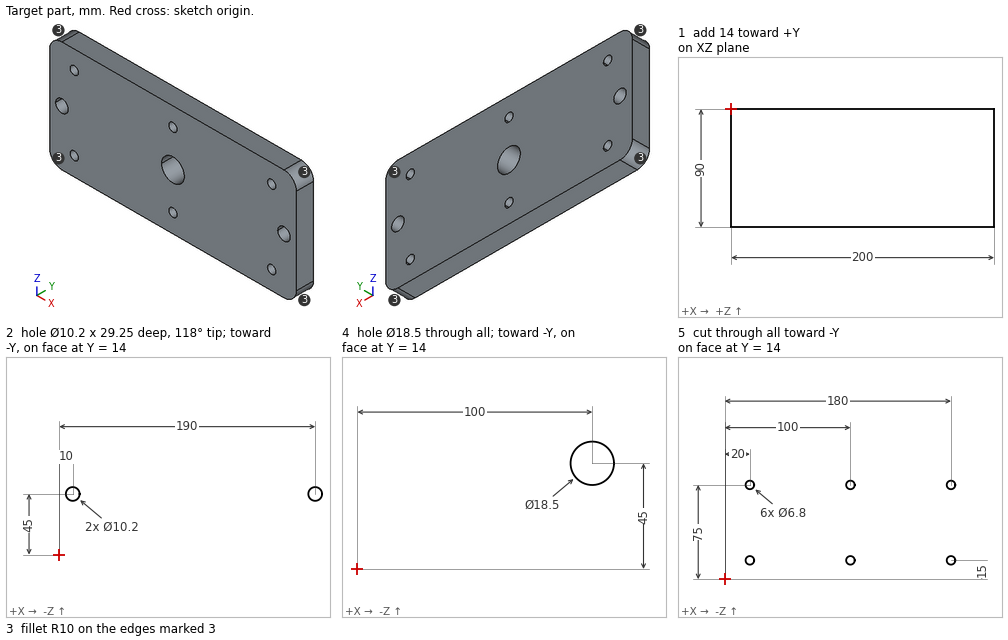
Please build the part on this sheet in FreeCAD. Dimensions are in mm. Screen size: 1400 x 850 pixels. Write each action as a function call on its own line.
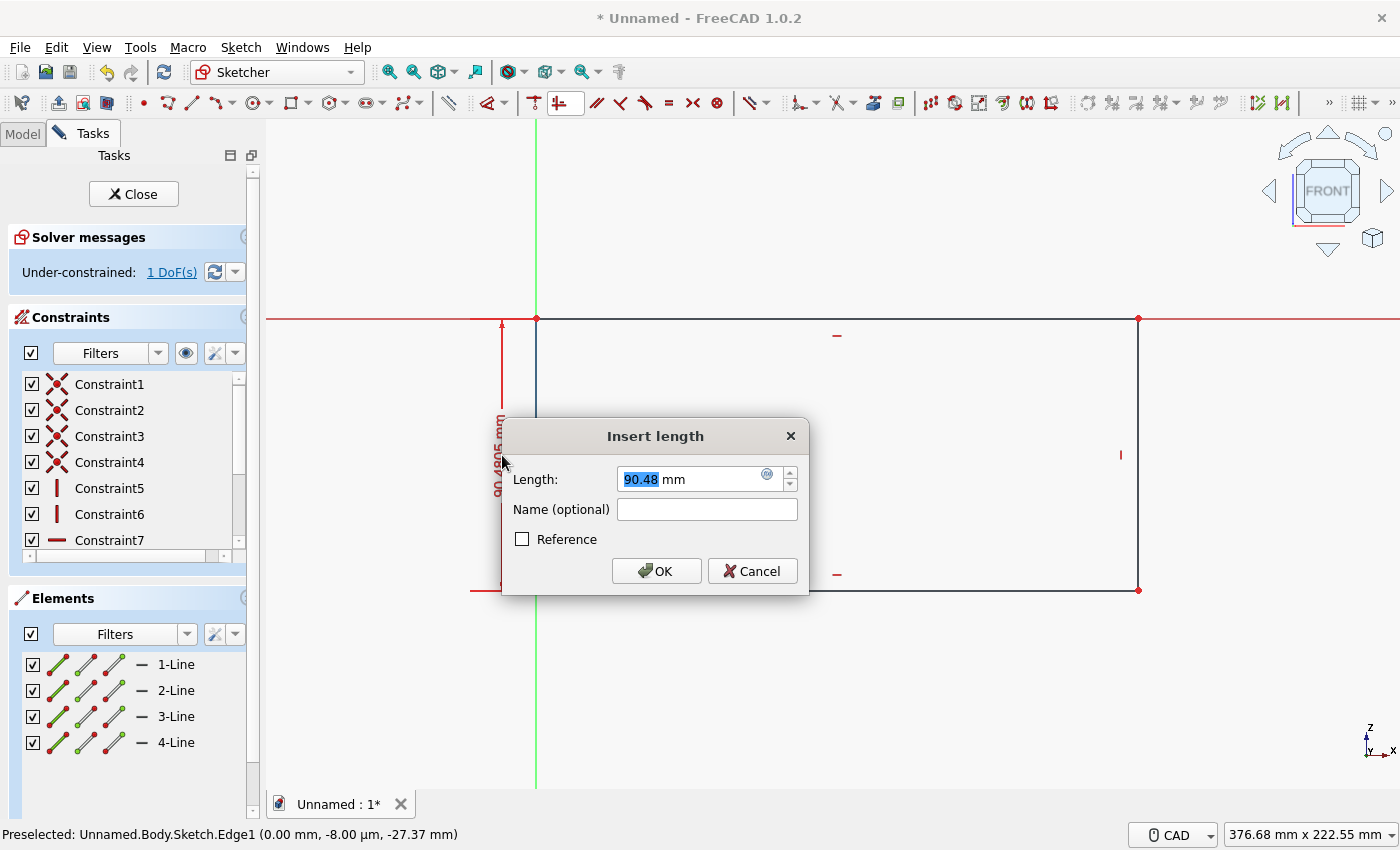
text(90)
key(Return)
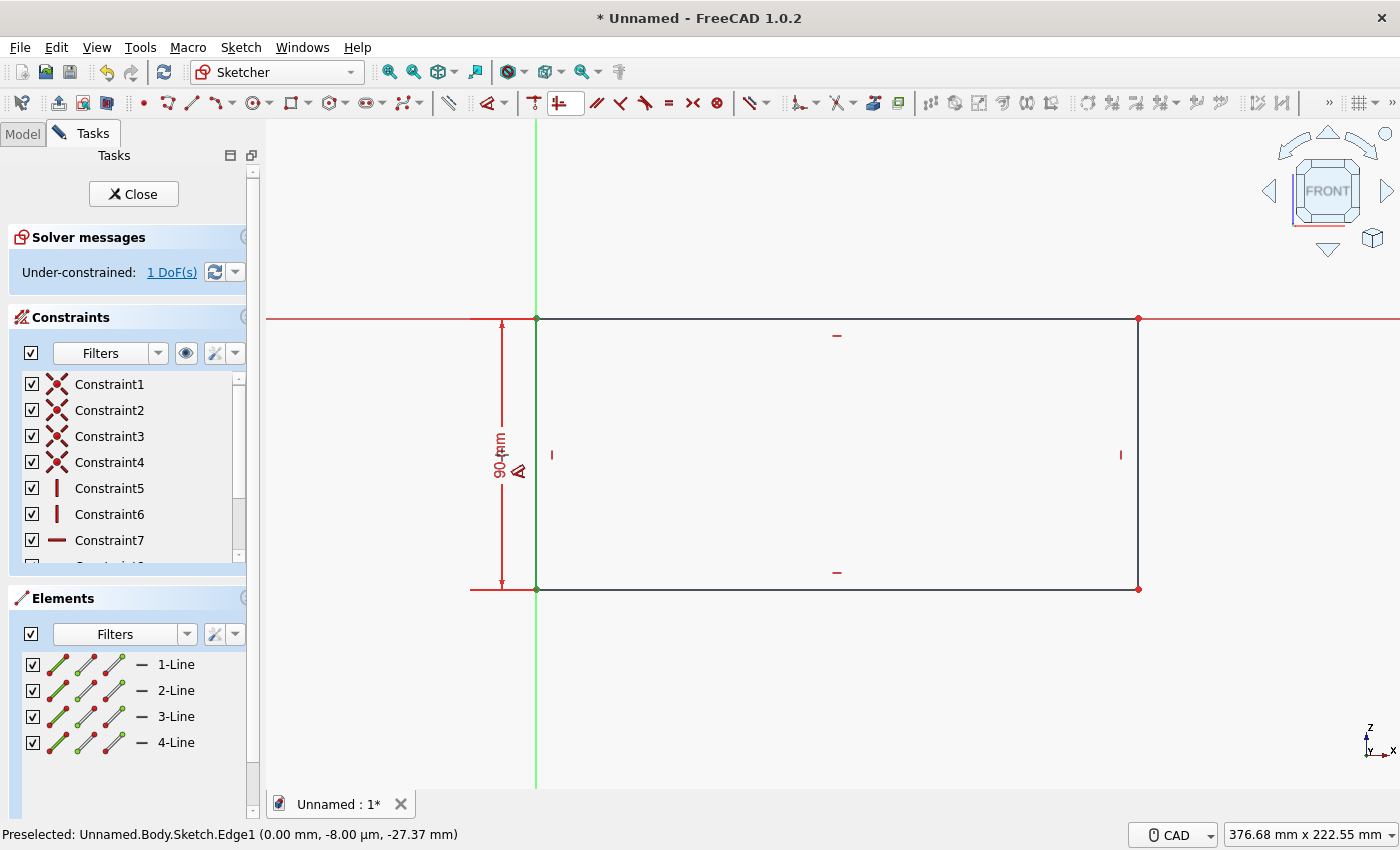
click(717, 590)
click(837, 624)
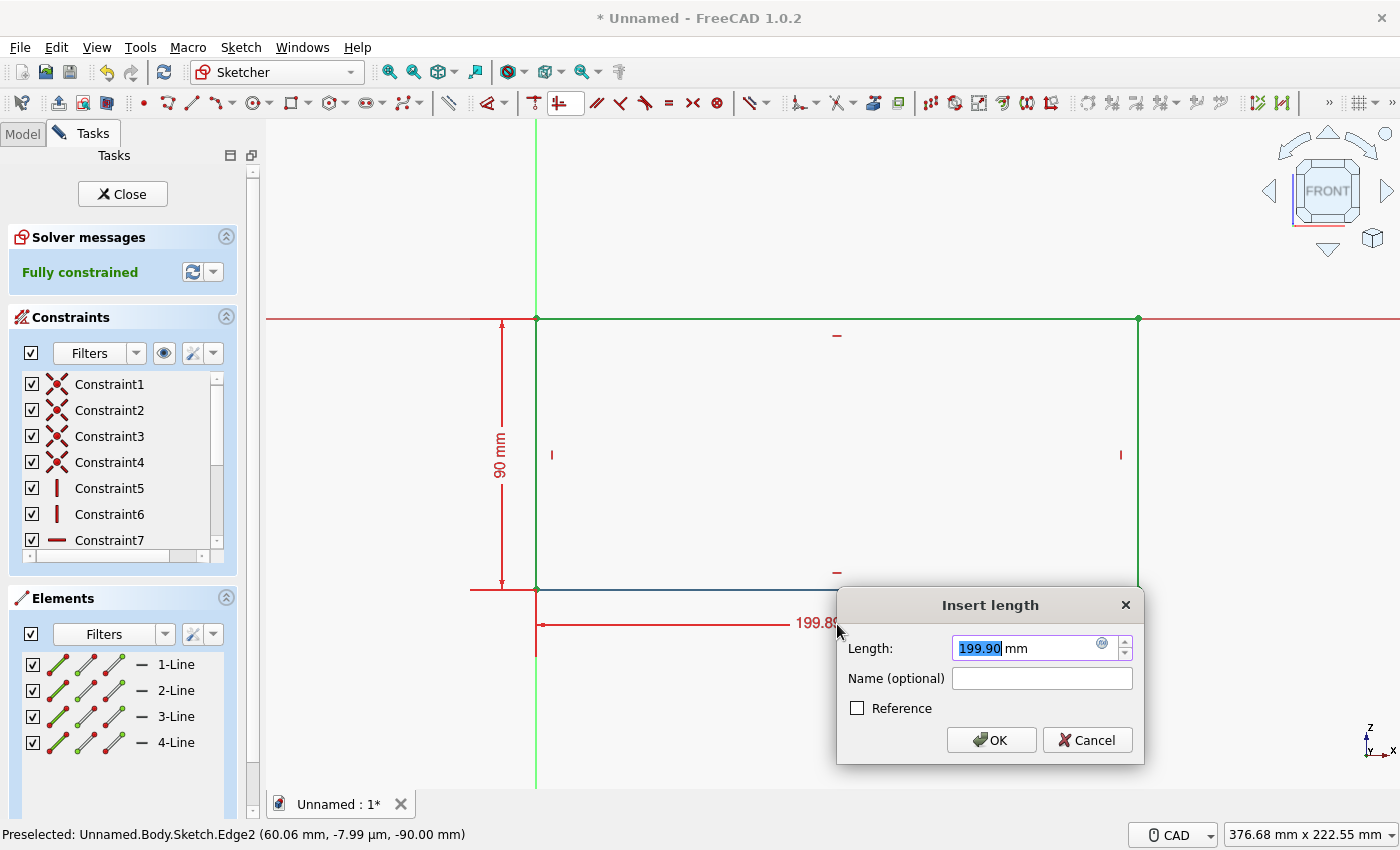
text(200)
key(Return)
key(Escape)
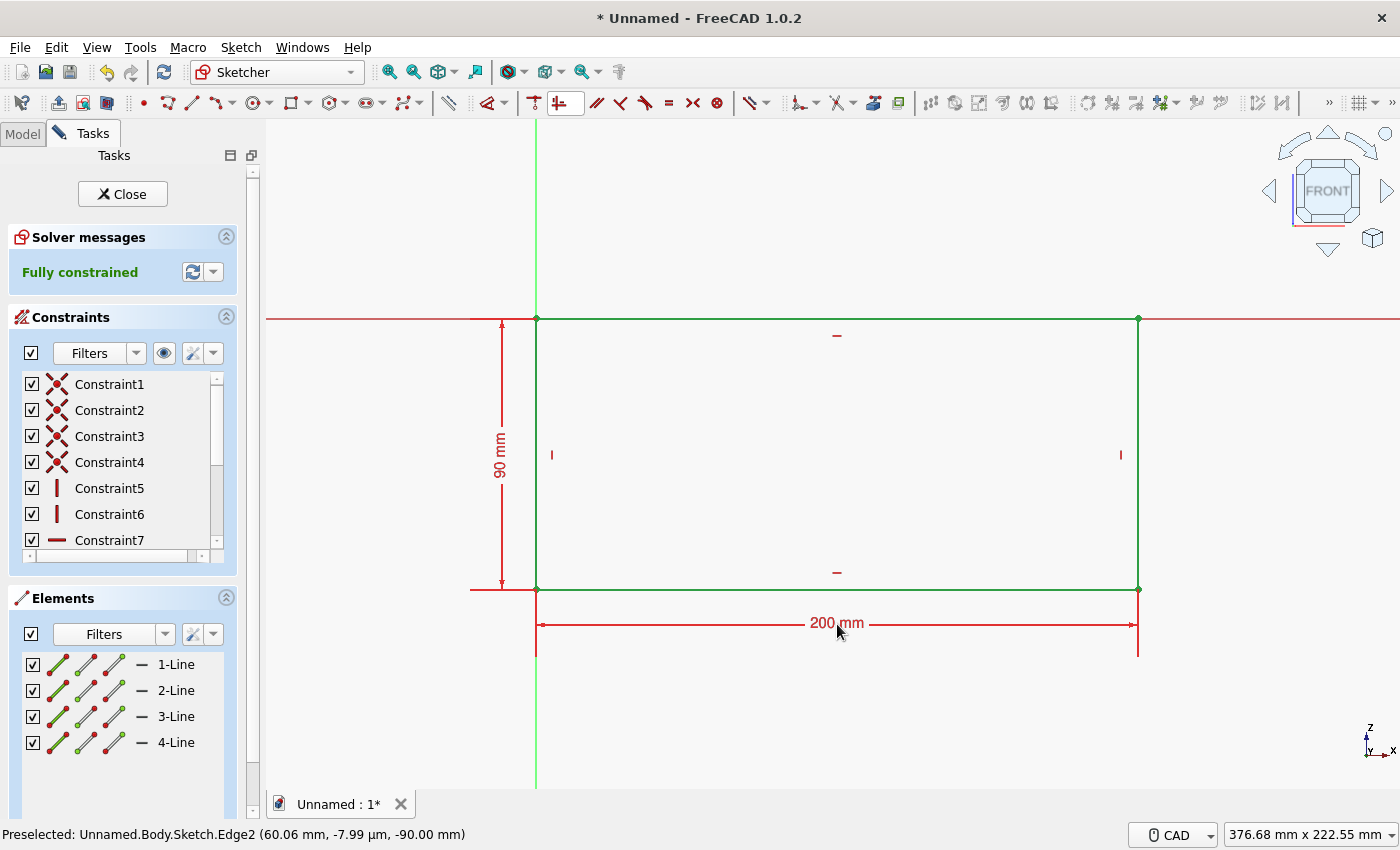
click(123, 194)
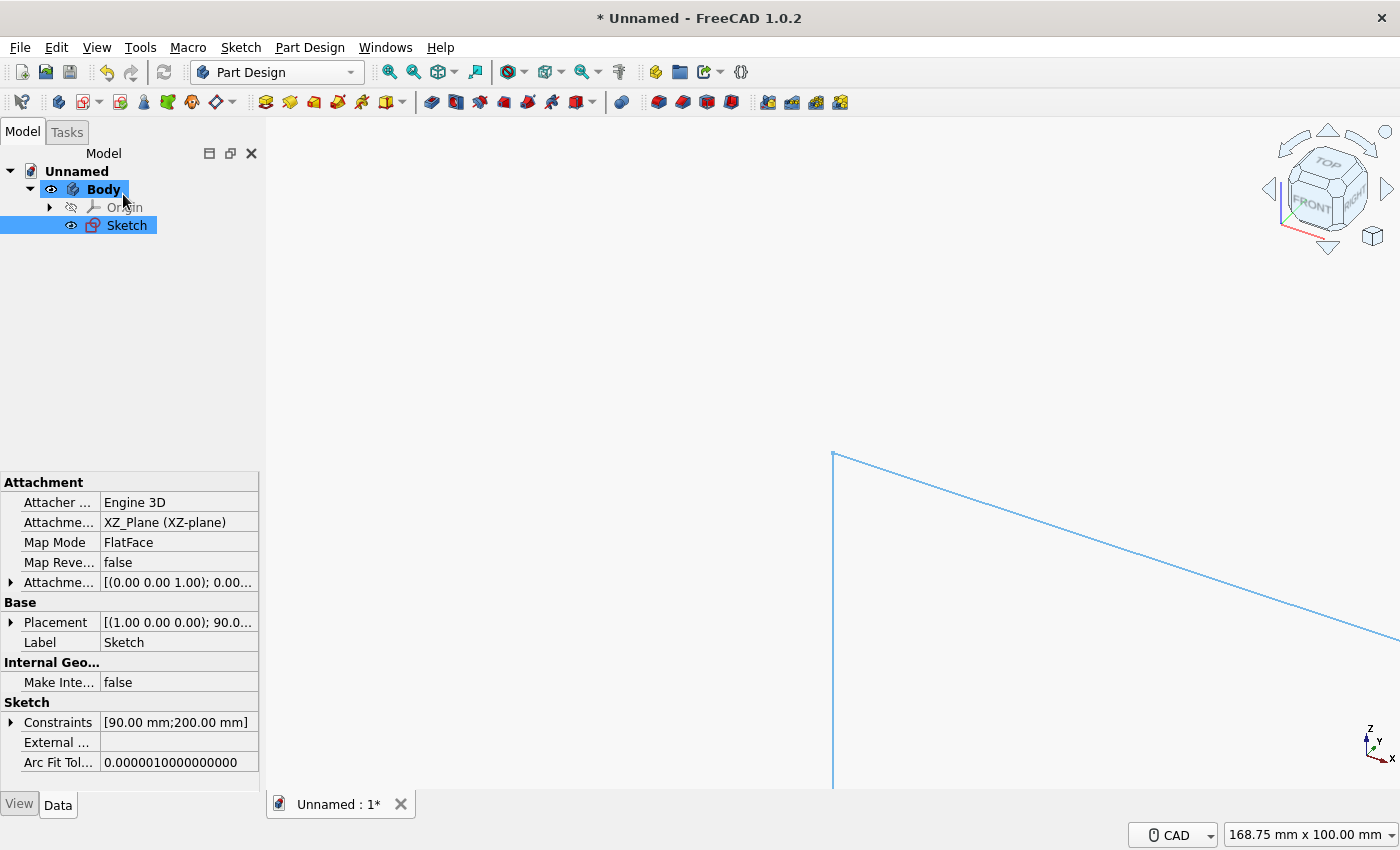
click(266, 102)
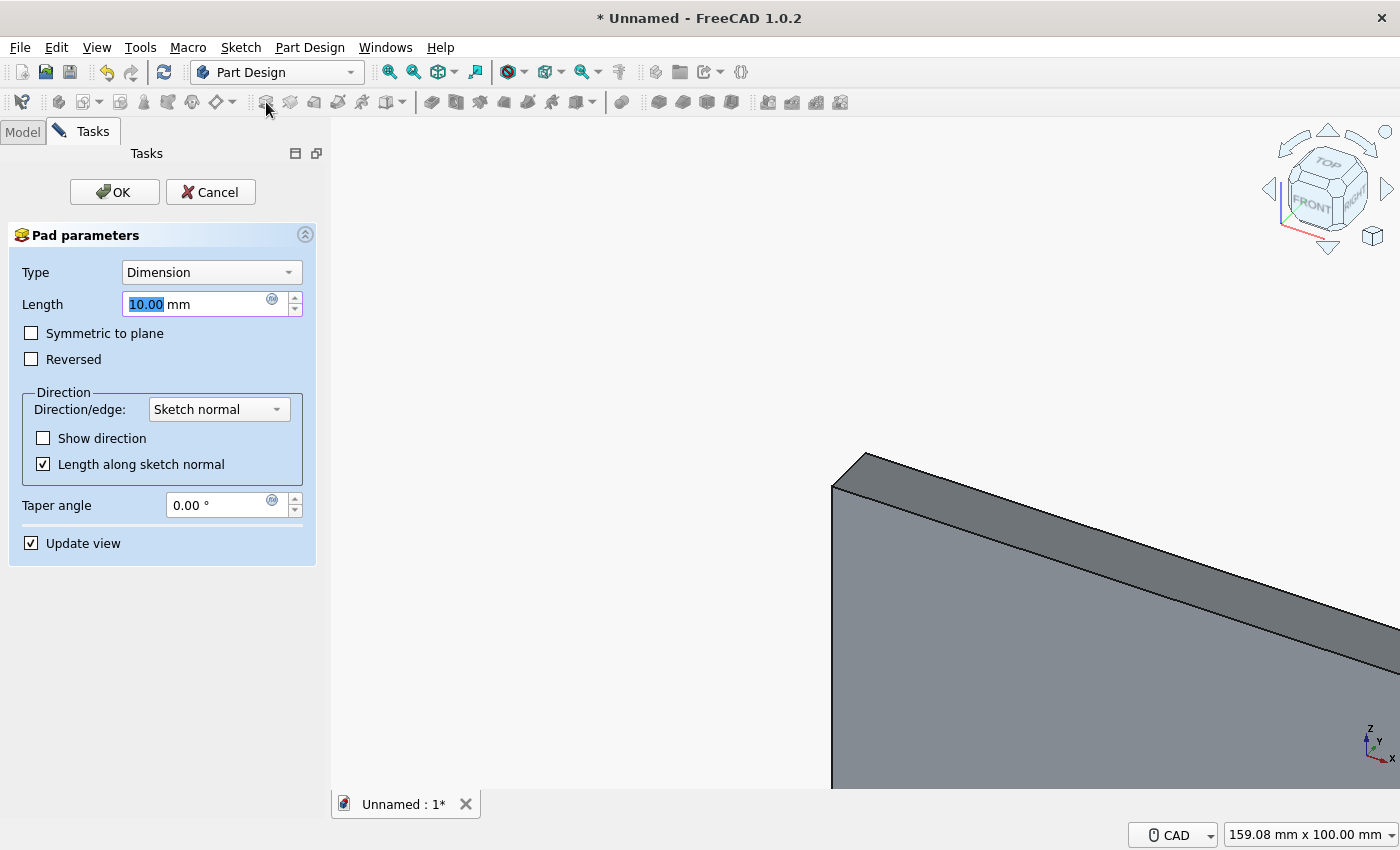
text(14)
key(Tab)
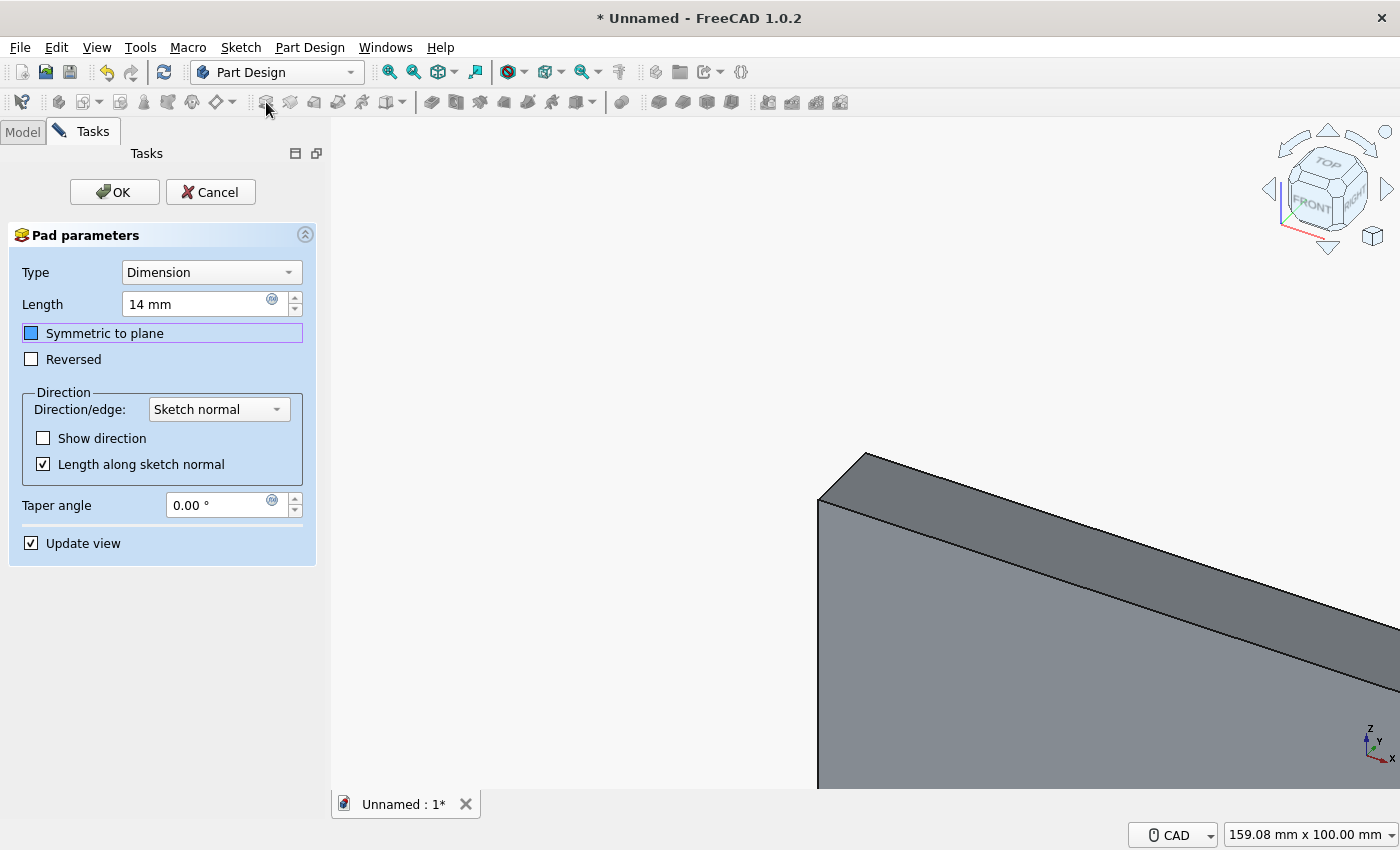
click(30, 359)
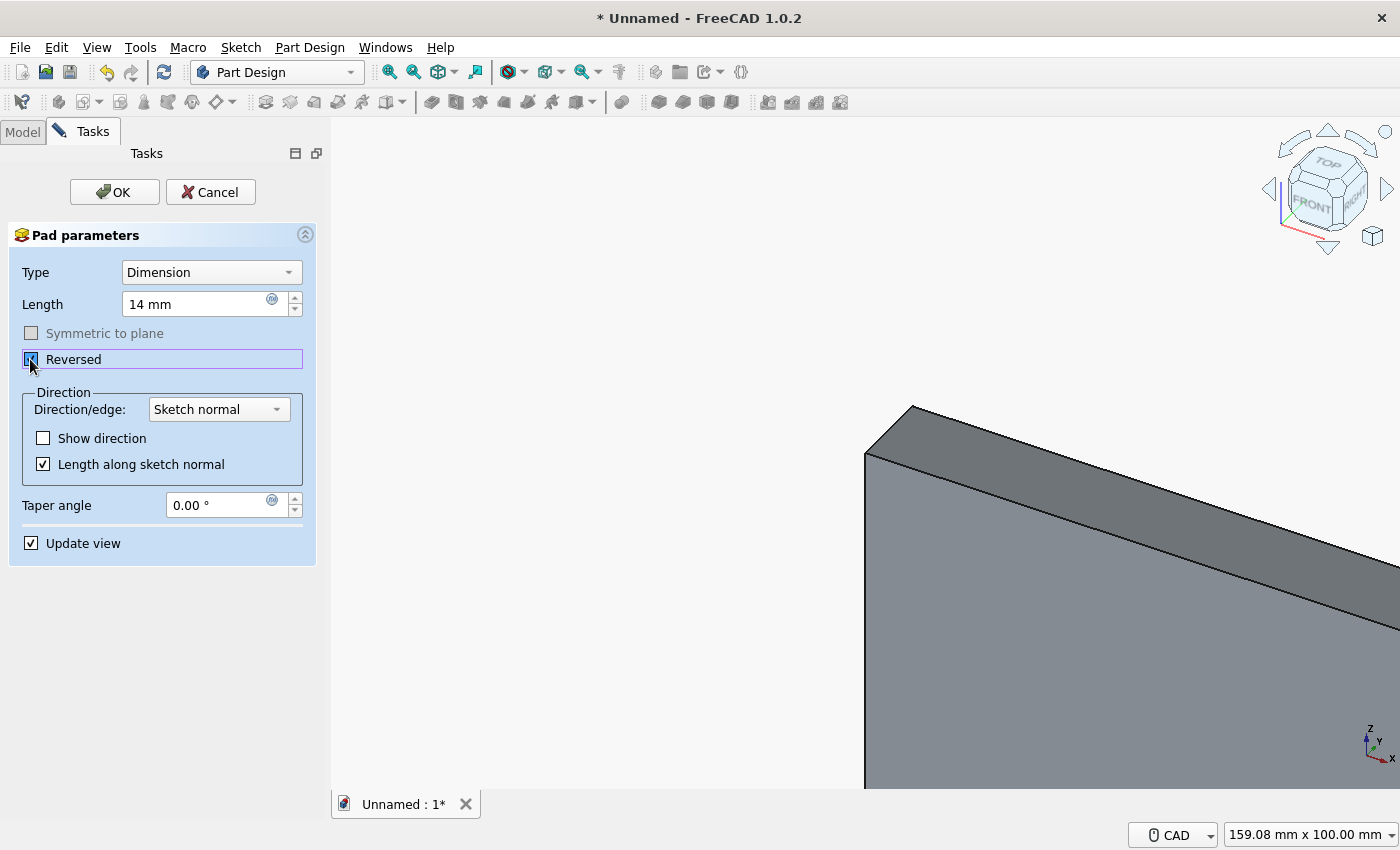
click(115, 192)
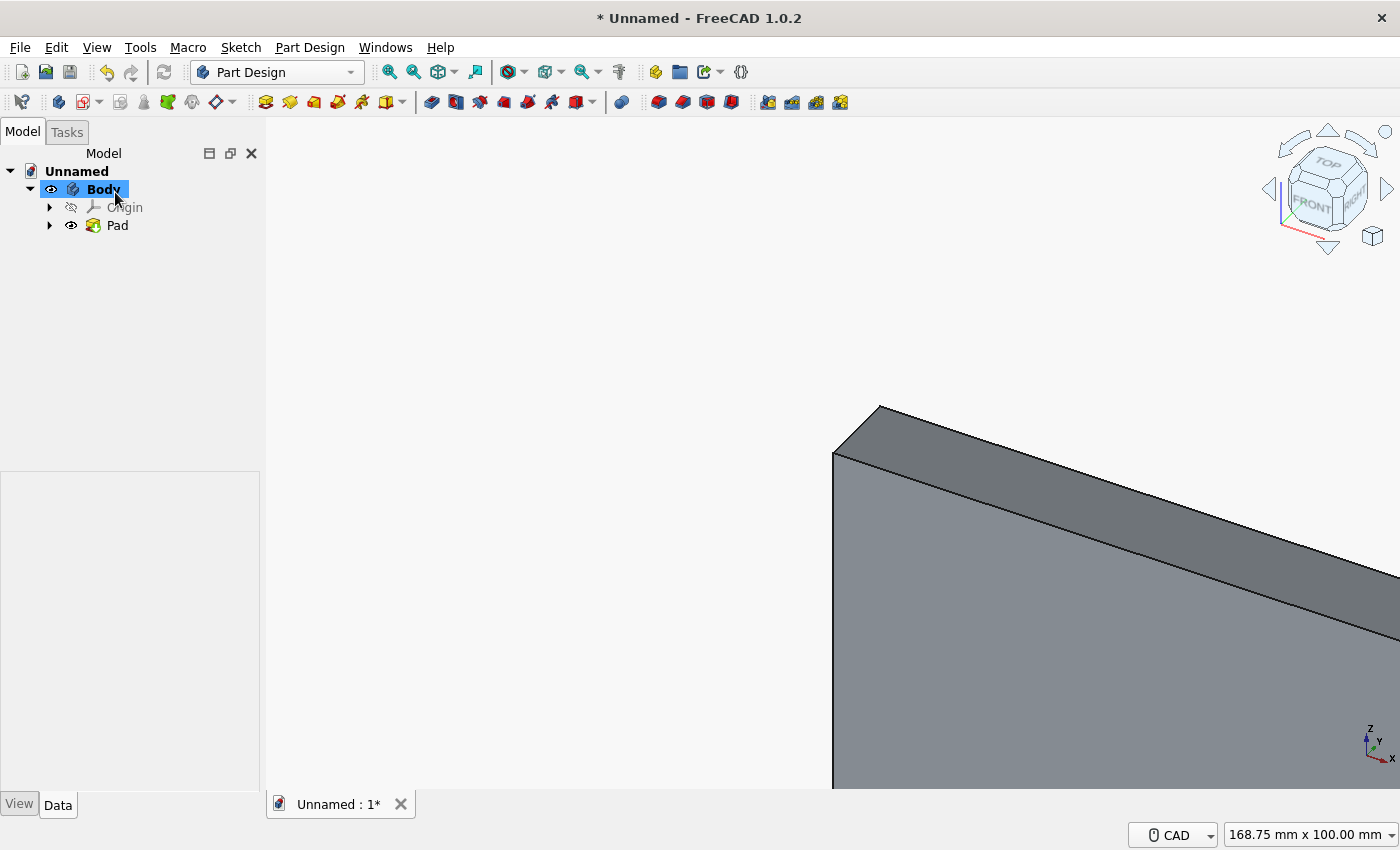
click(390, 72)